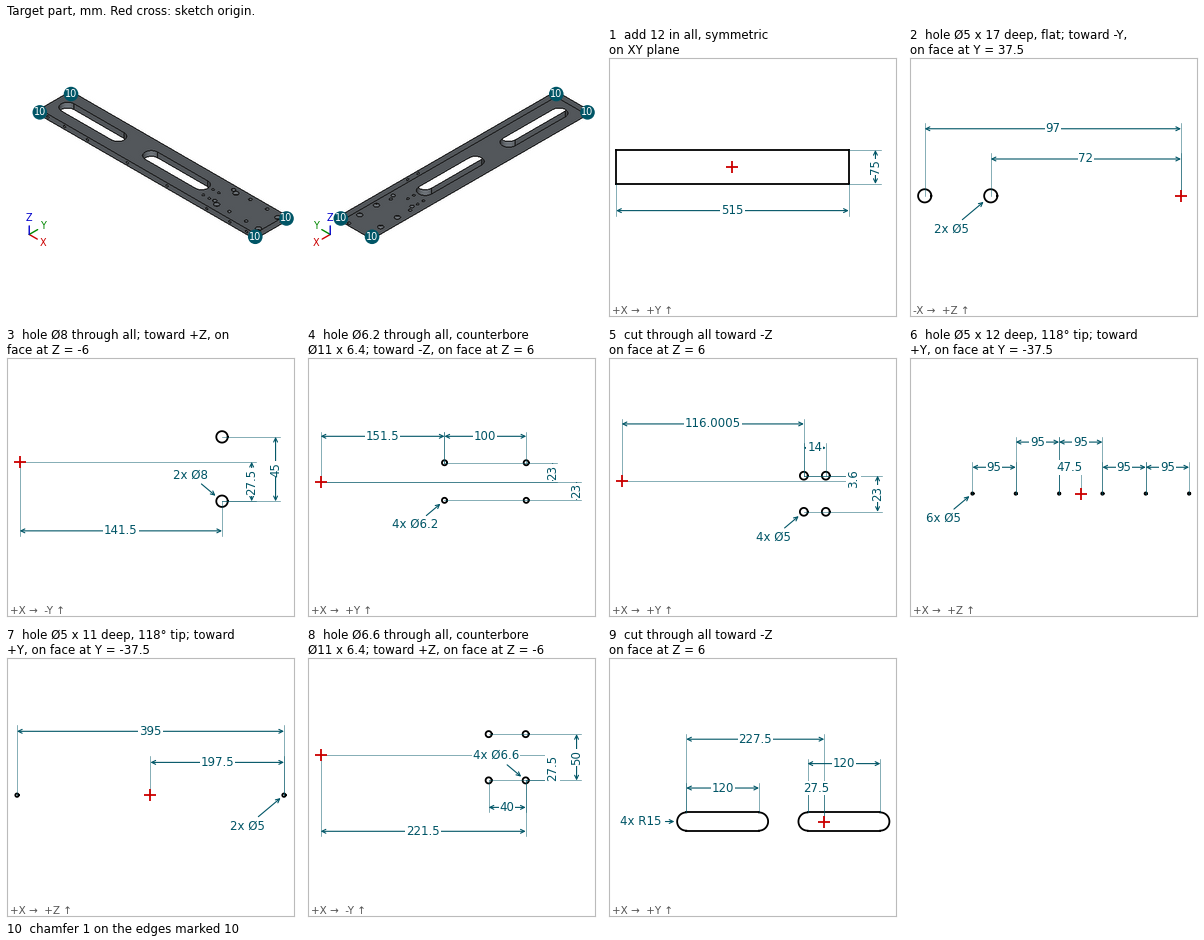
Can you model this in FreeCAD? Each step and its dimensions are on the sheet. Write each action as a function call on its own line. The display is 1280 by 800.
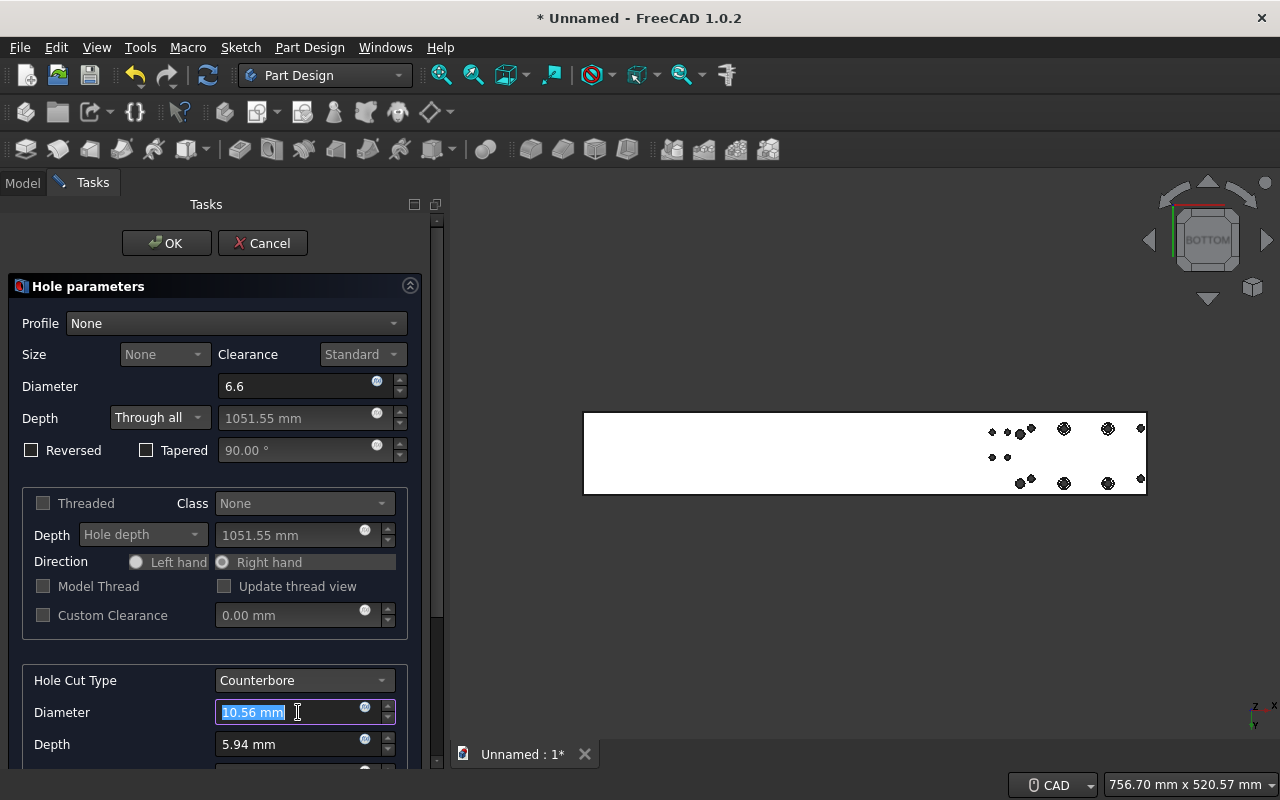
text(11)
key(Tab)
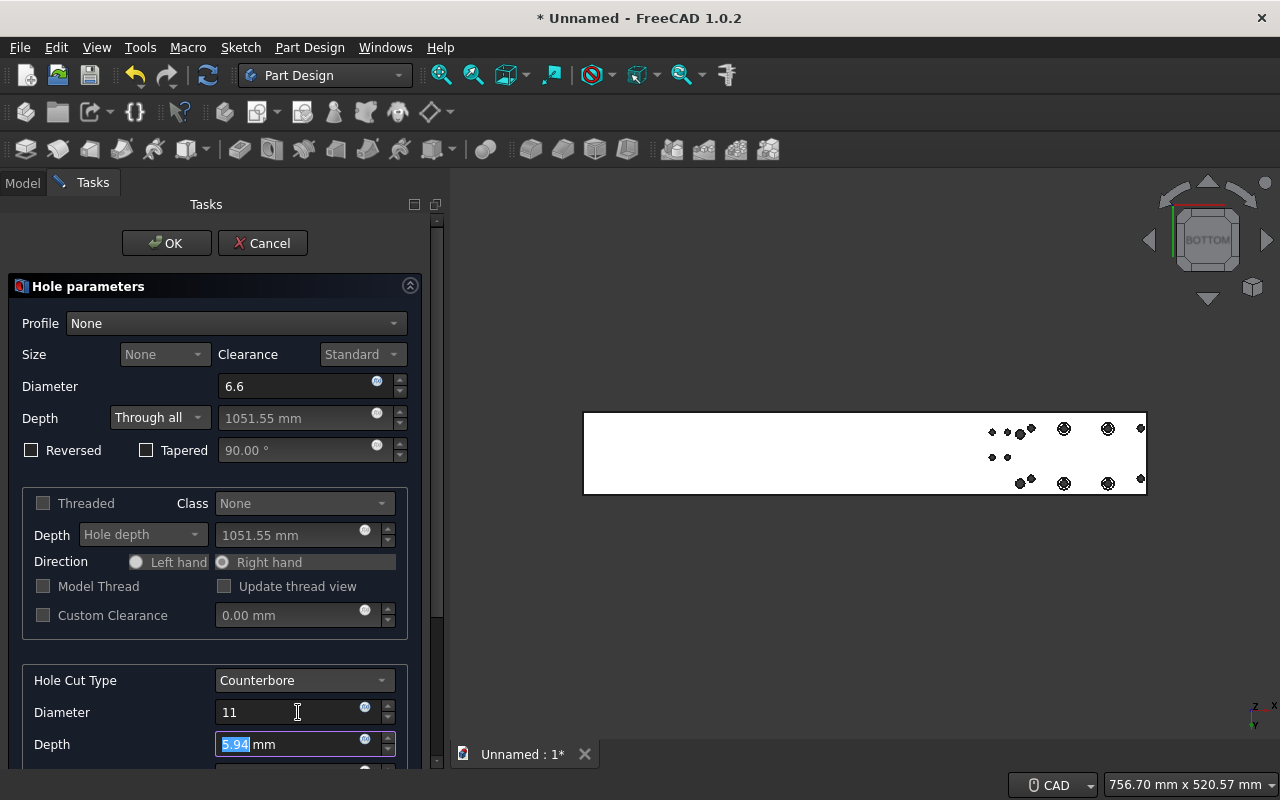
text(6.4)
key(Tab)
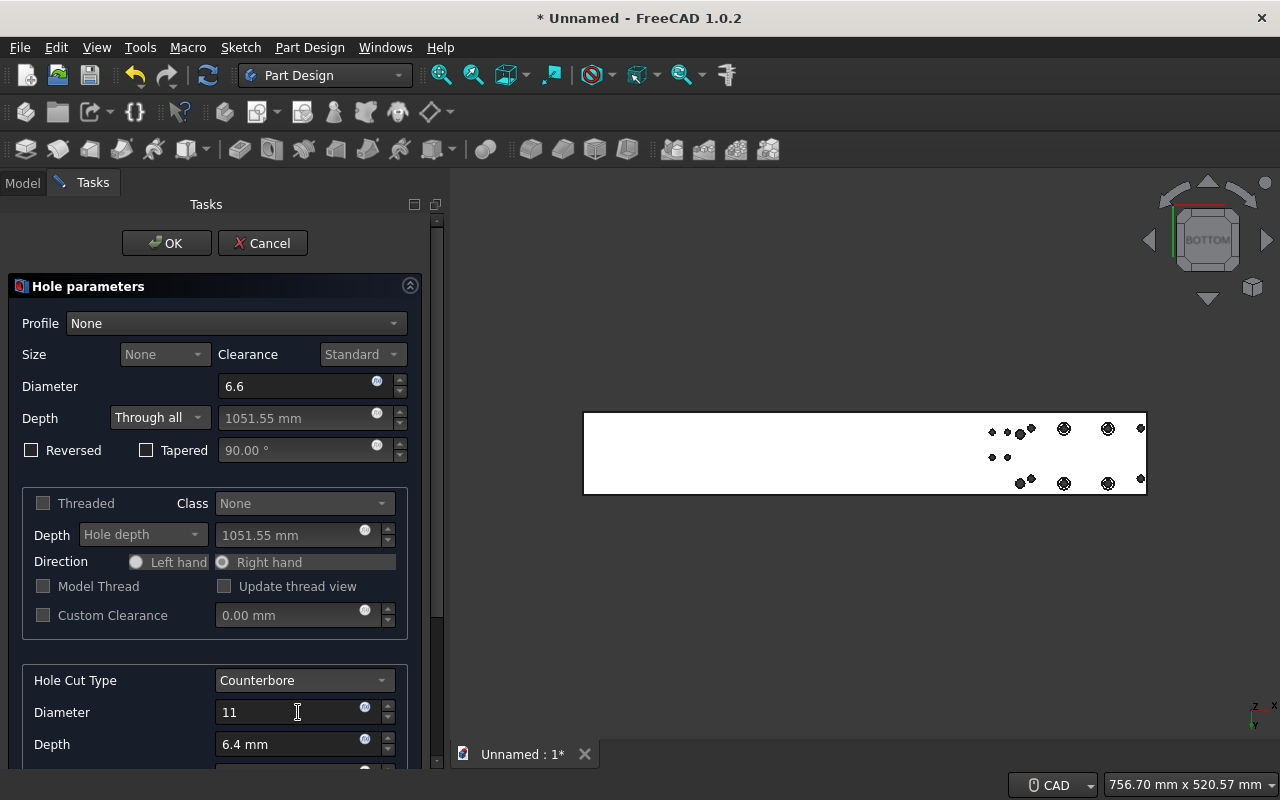
click(167, 243)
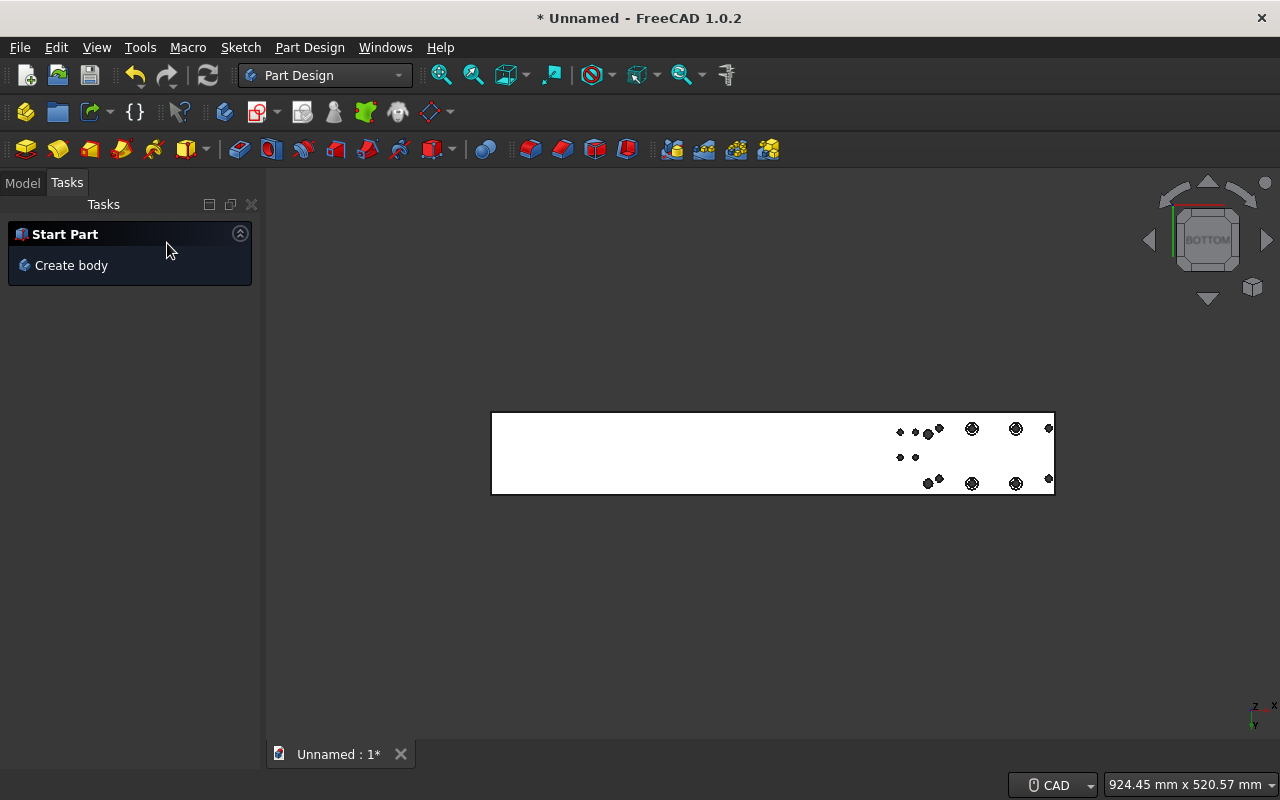
key(0)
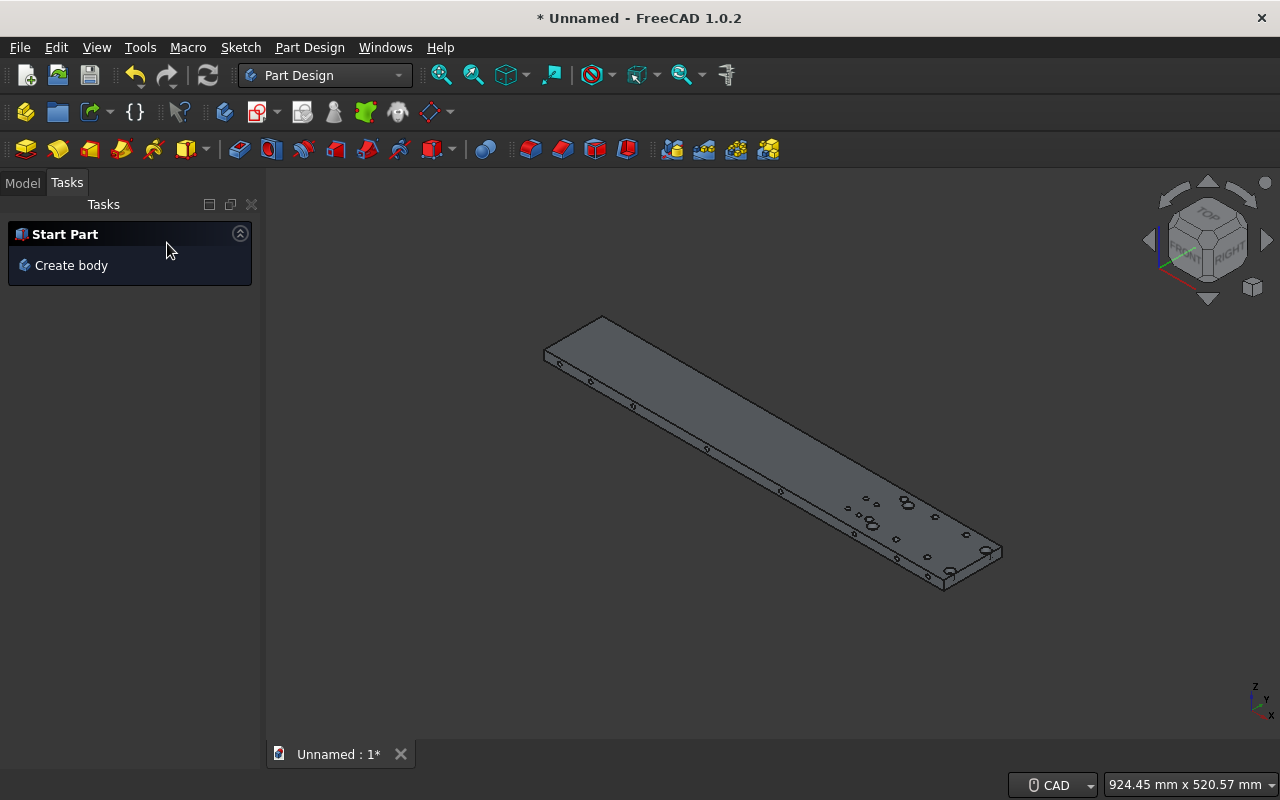
click(830, 480)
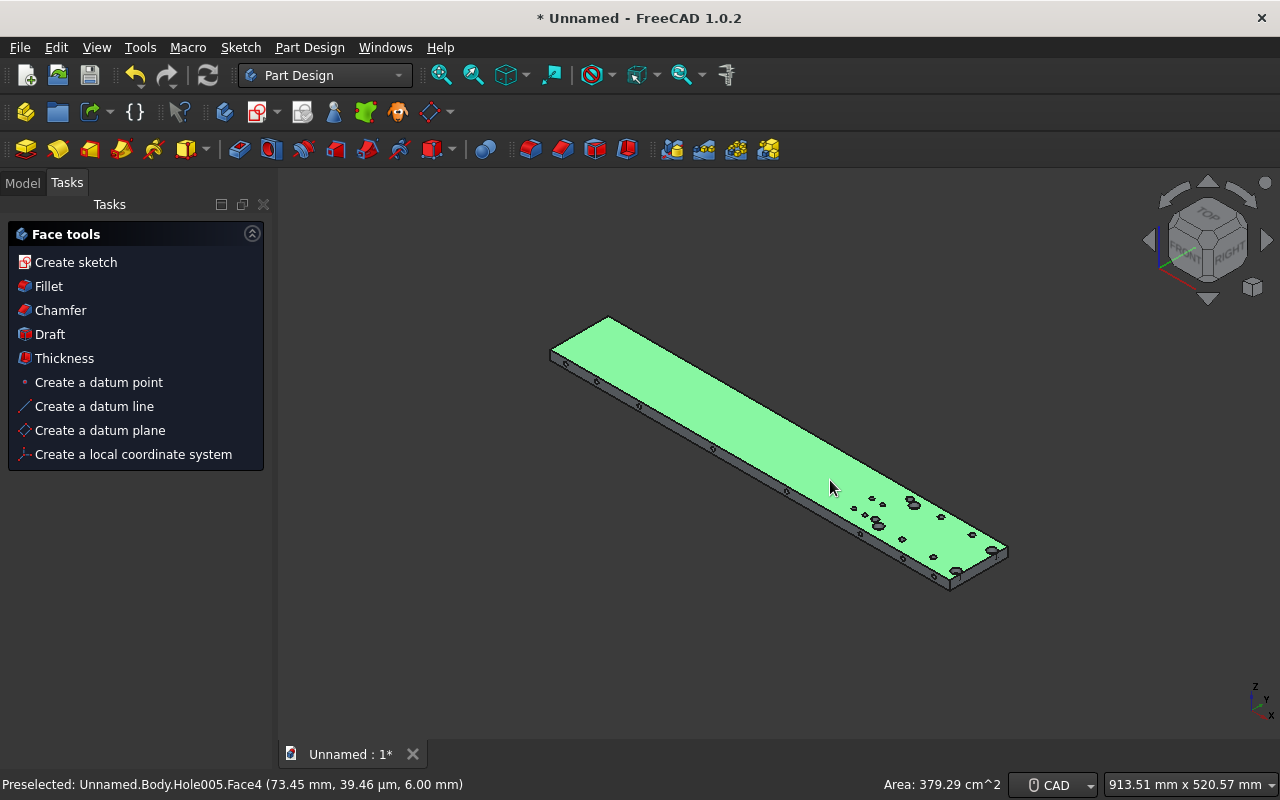
click(258, 112)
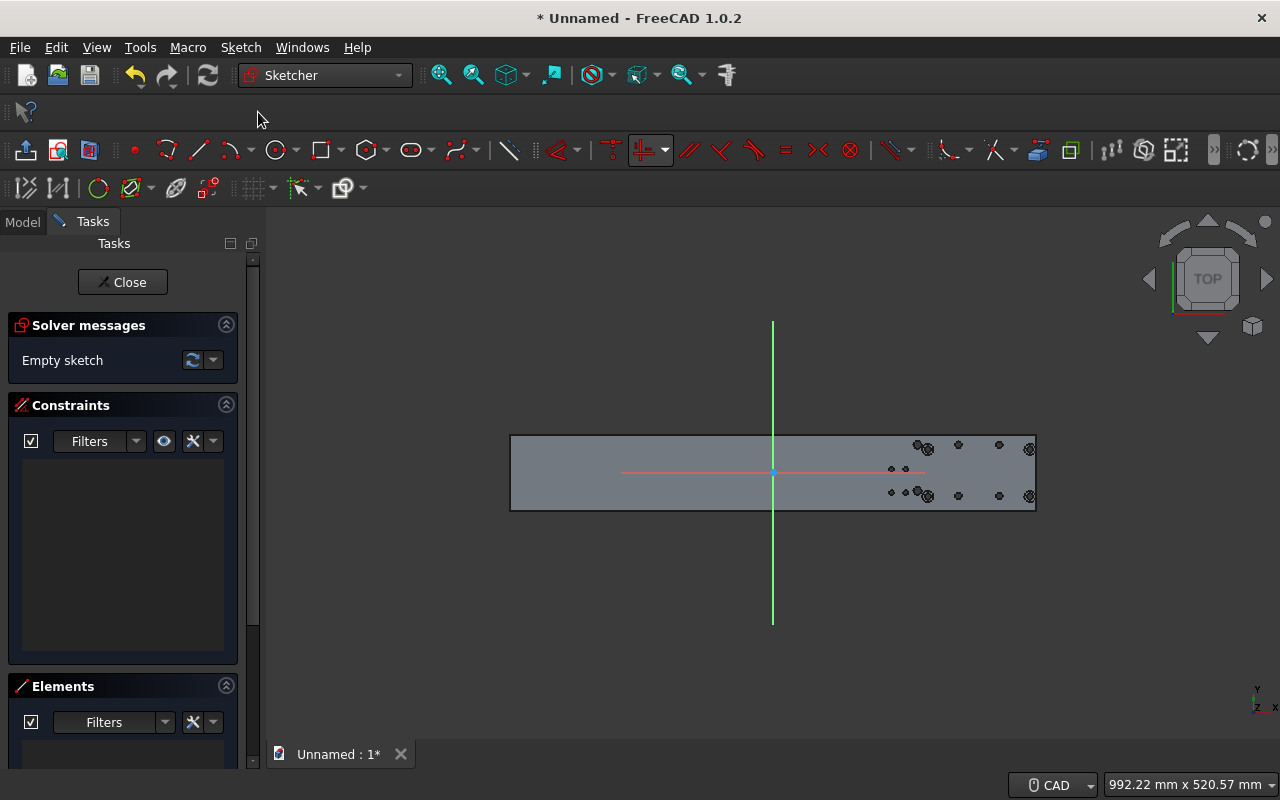
scroll(703, 473, up, 2)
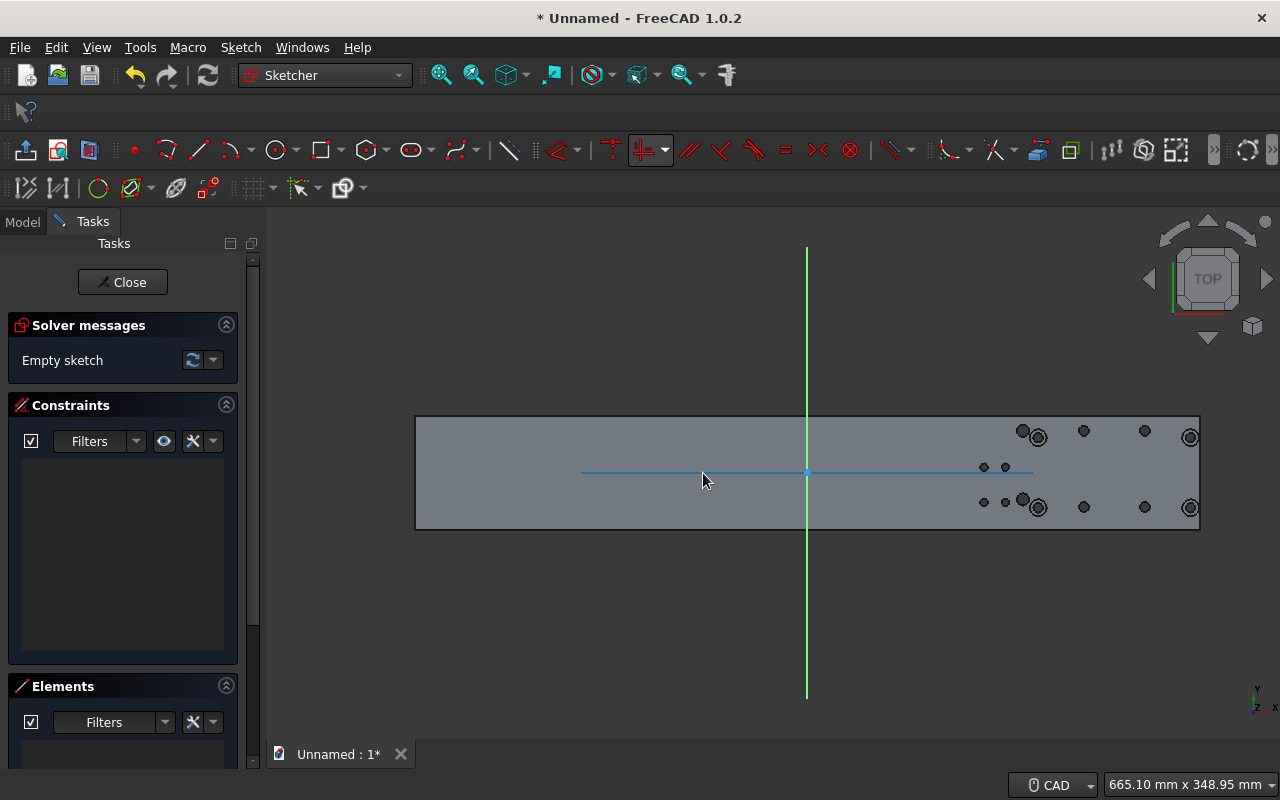
key(g)
key(s)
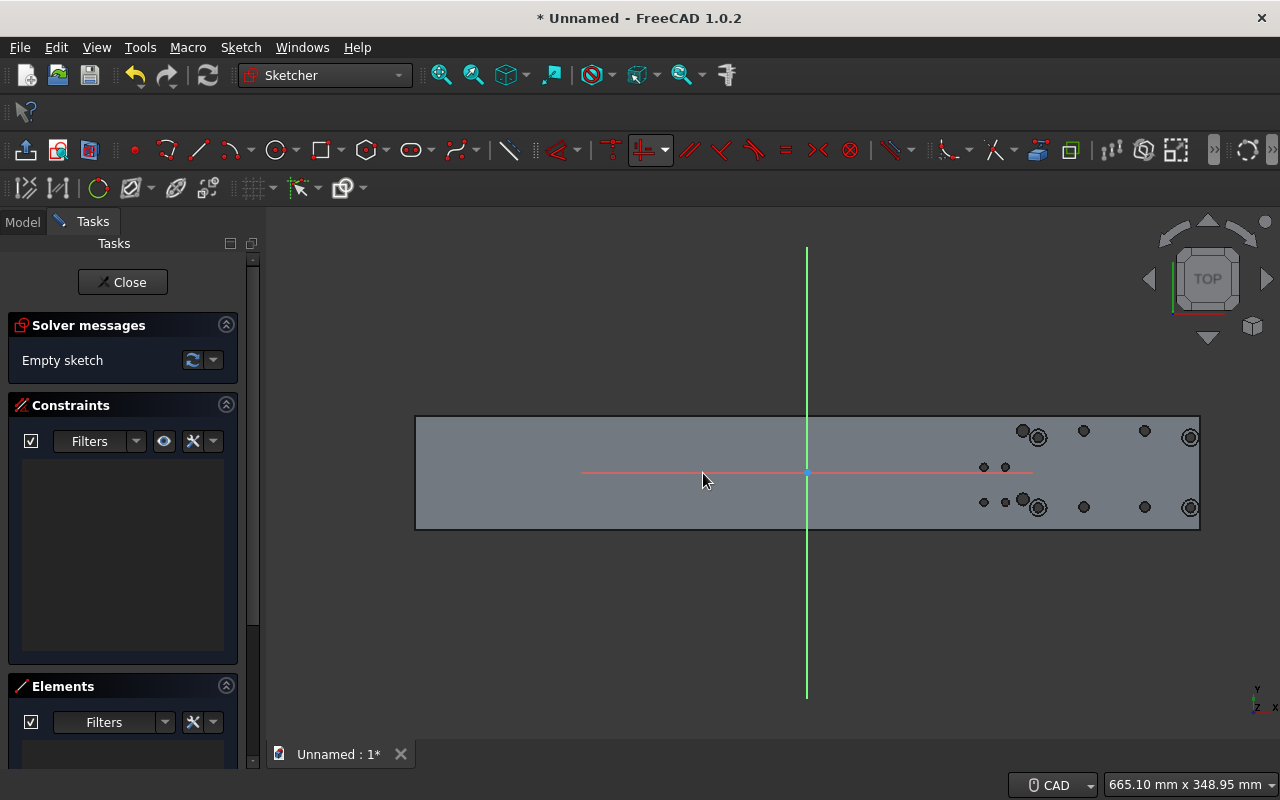
click(460, 473)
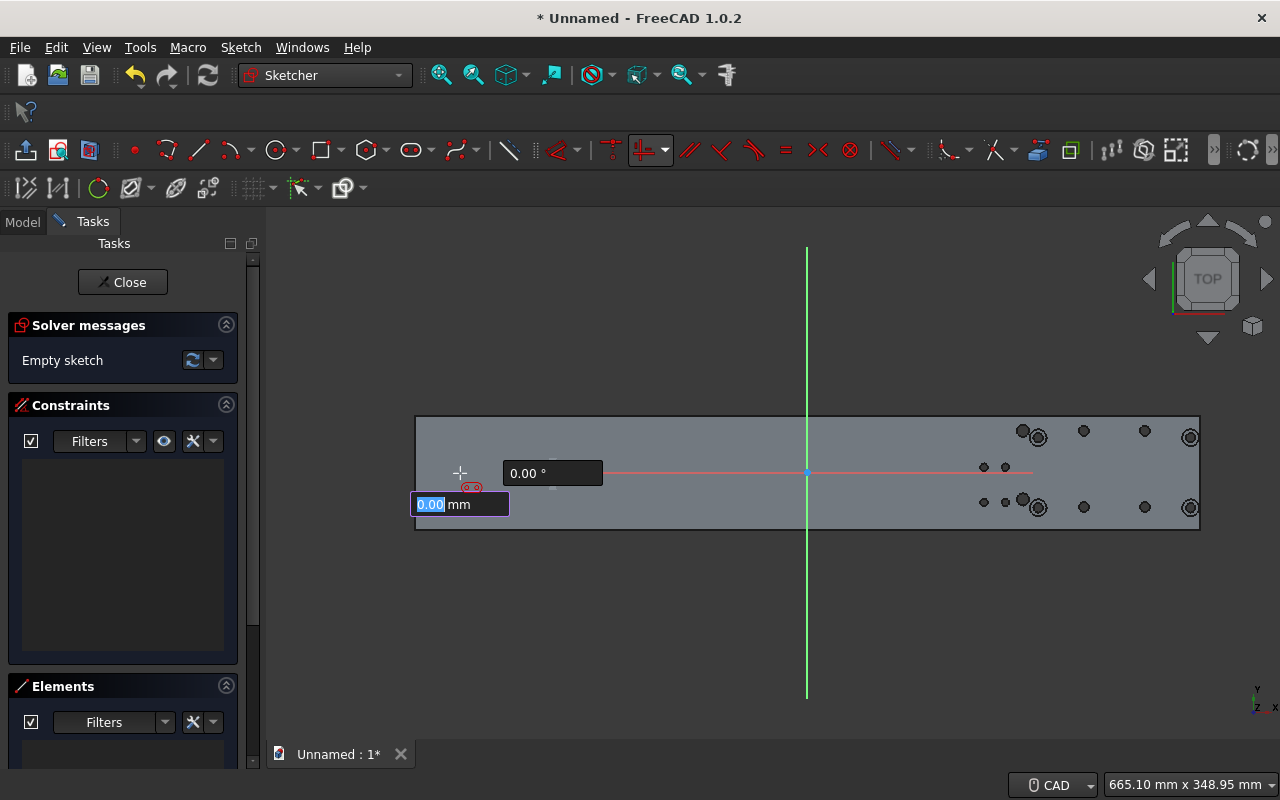
click(643, 464)